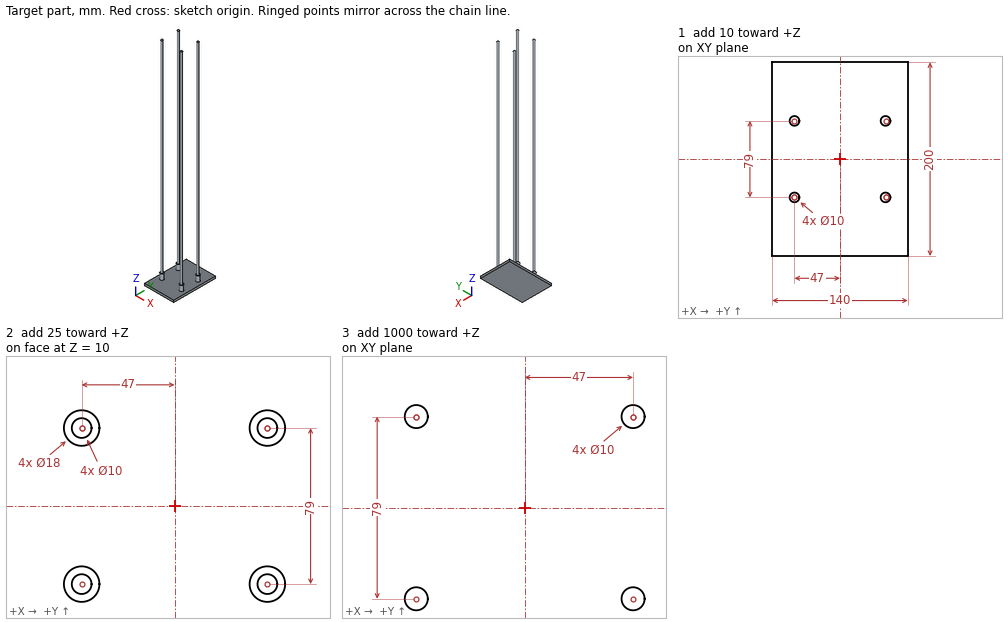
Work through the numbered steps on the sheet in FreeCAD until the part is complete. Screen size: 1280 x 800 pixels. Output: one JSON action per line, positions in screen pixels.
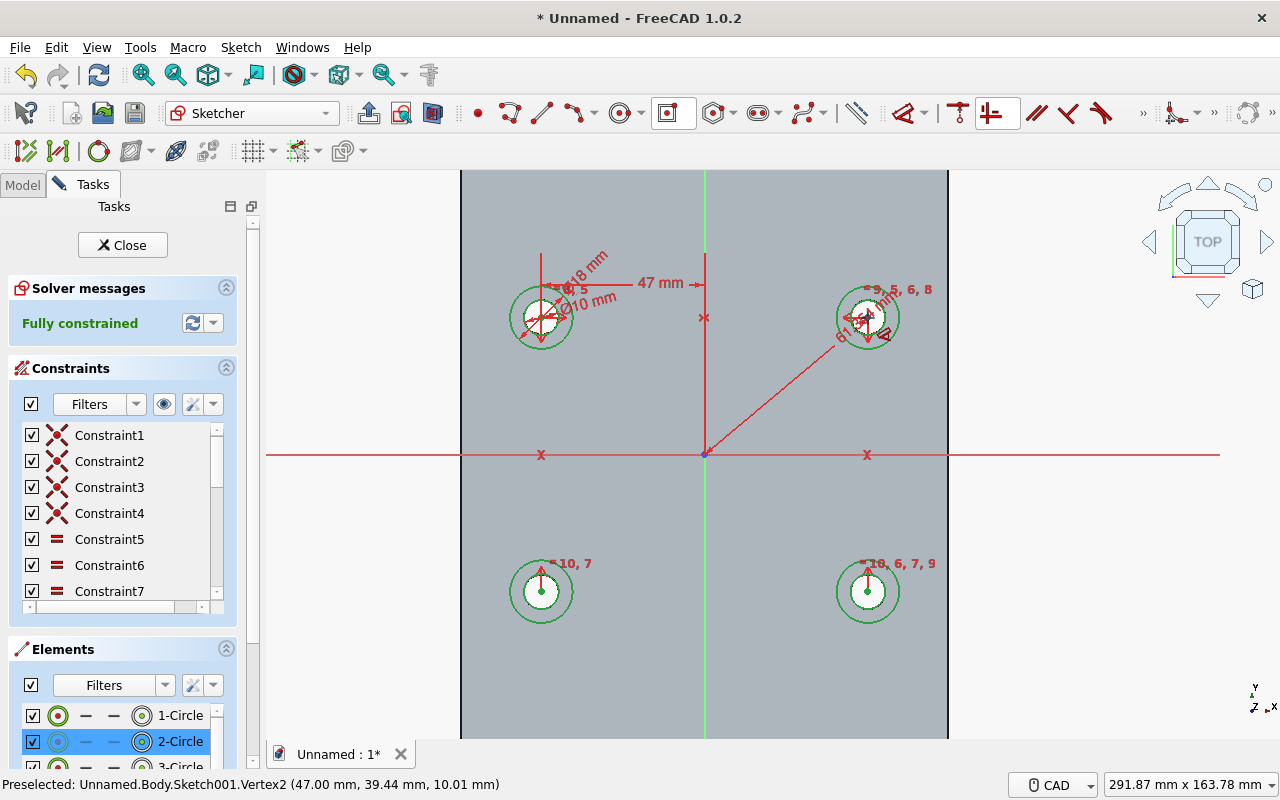
{"action": "left_click", "coordinate": [868, 592]}
{"action": "left_click", "coordinate": [902, 392]}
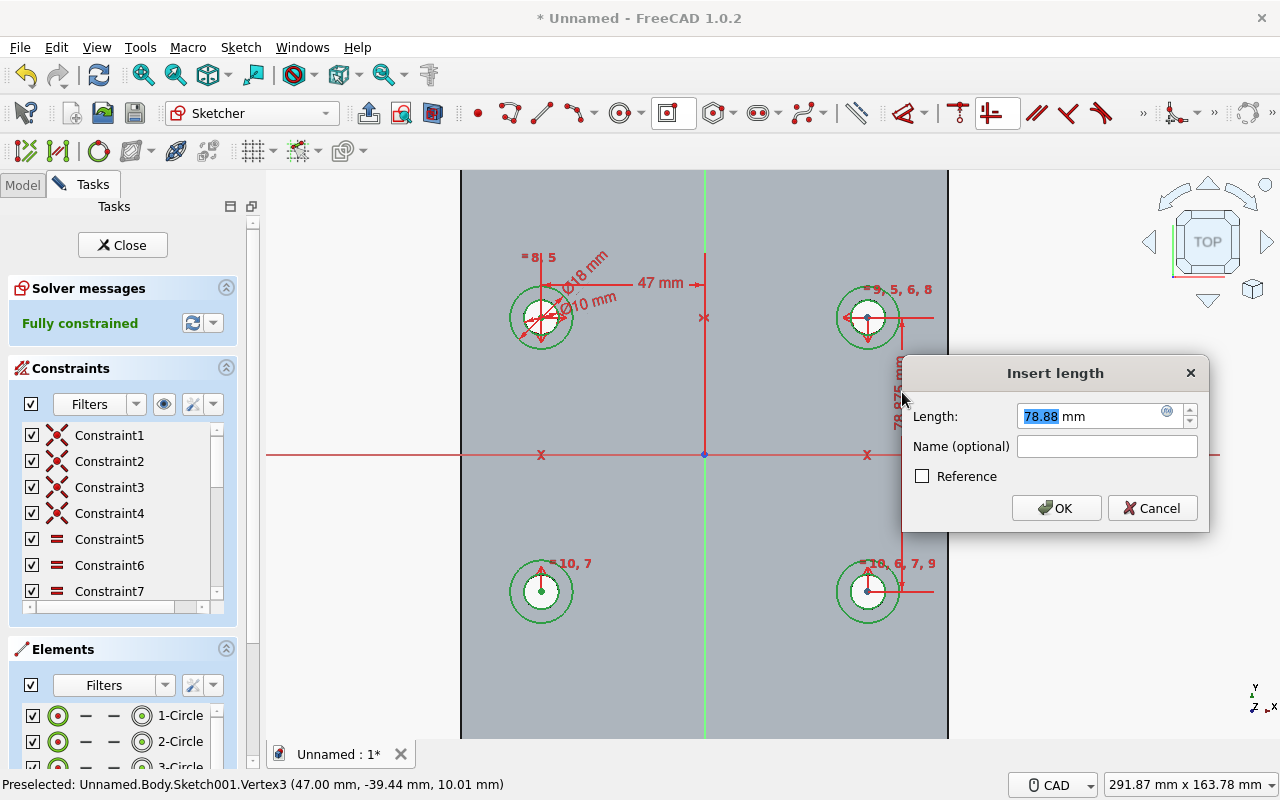
{"action": "type", "text": "79"}
{"action": "key", "text": "Return"}
{"action": "key", "text": "Escape"}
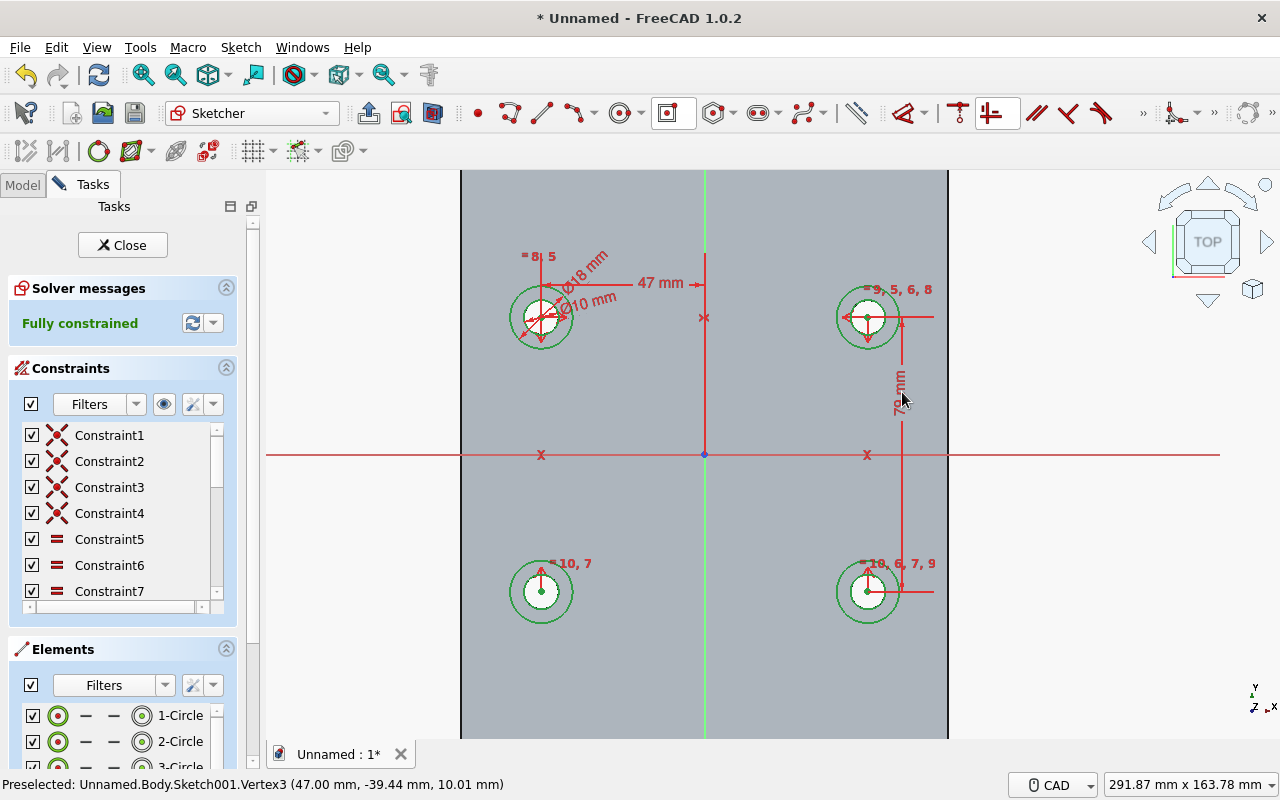
{"action": "left_click", "coordinate": [123, 245]}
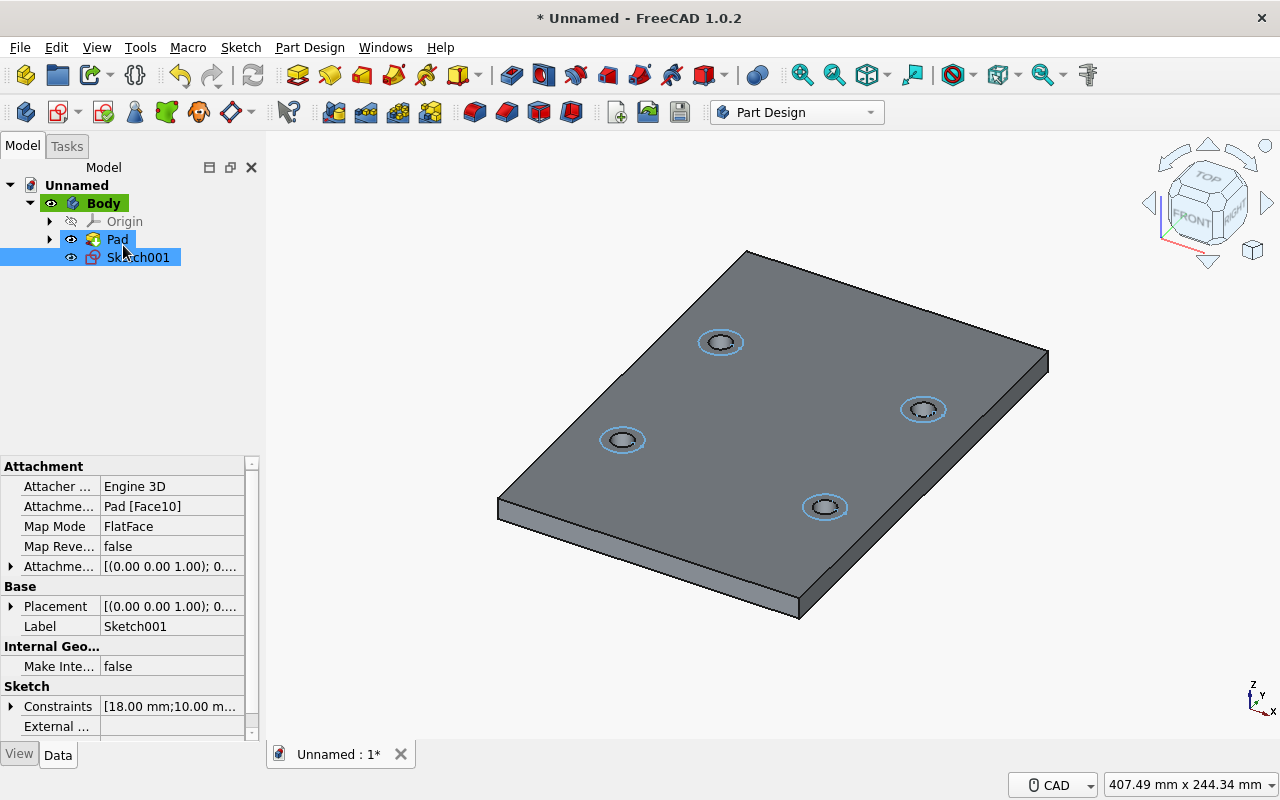
{"action": "left_click", "coordinate": [298, 76]}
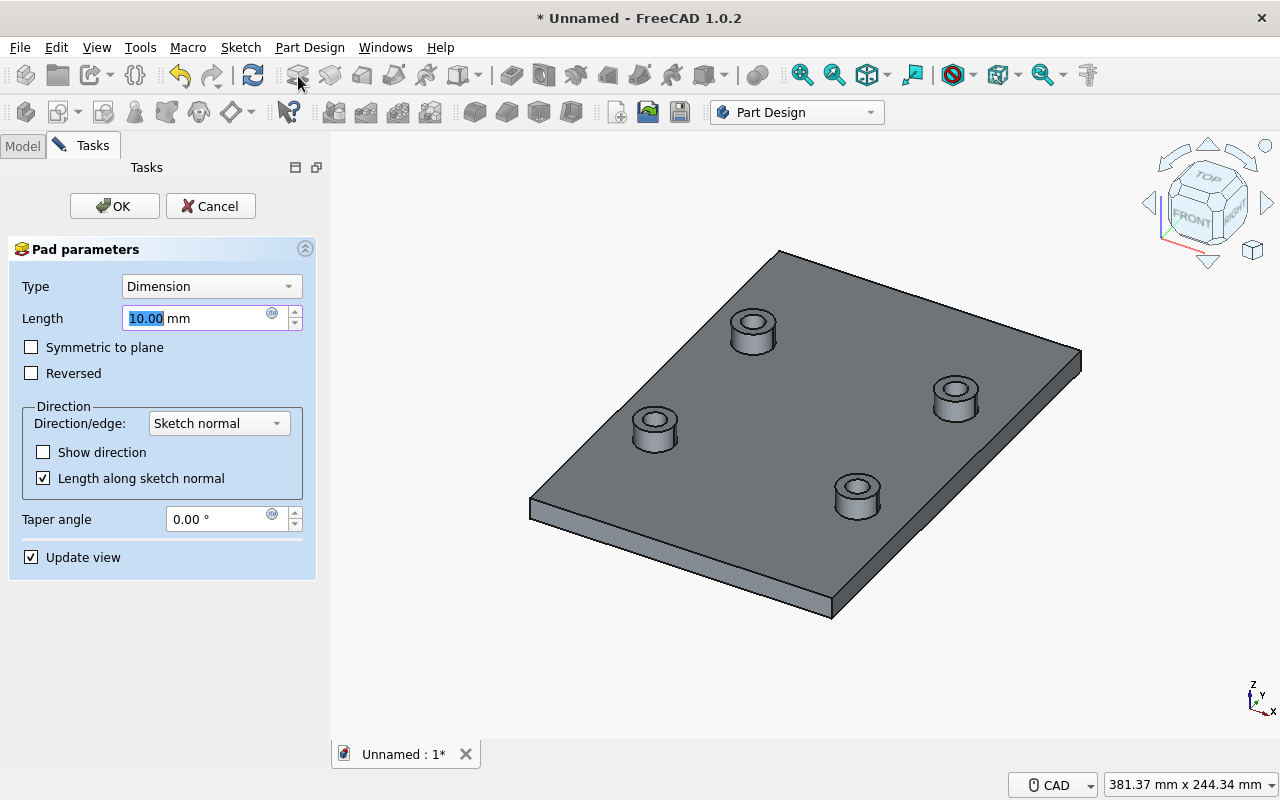
{"action": "type", "text": "25"}
{"action": "key", "text": "Tab"}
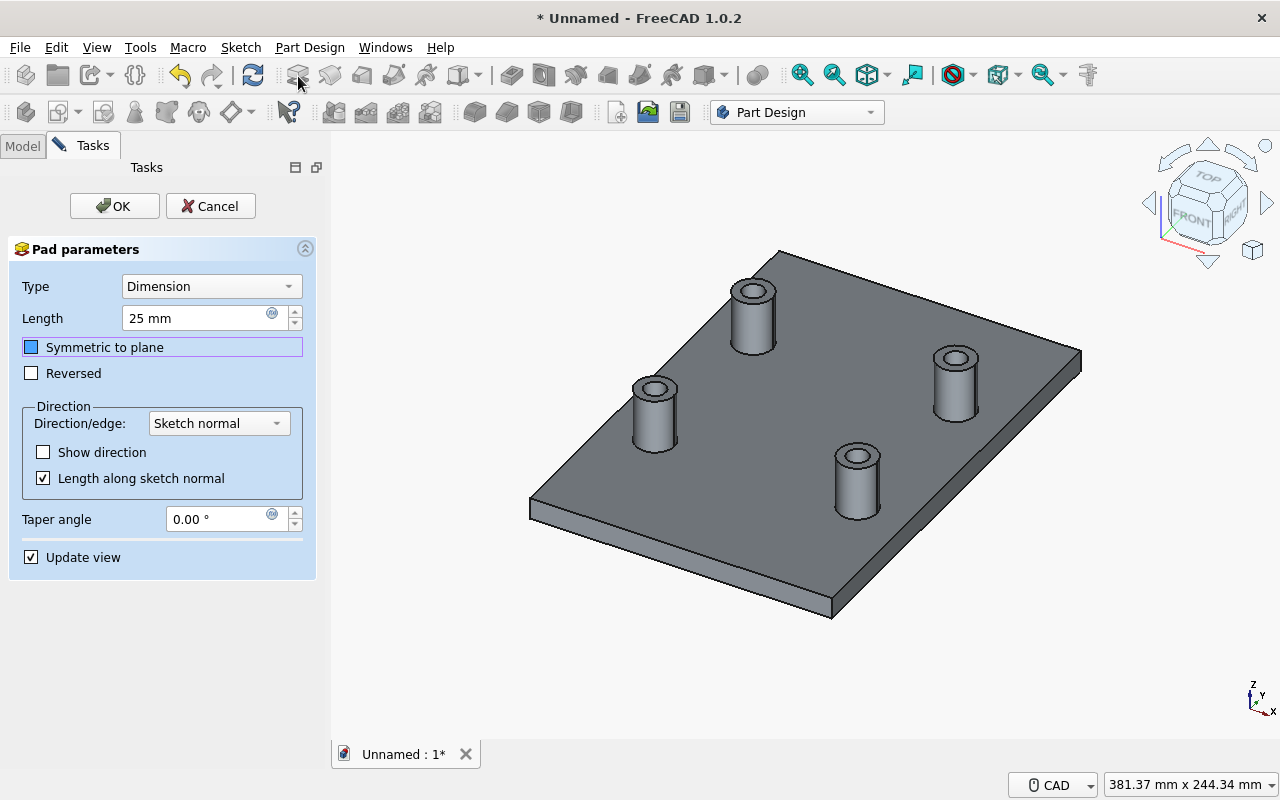
{"action": "left_click", "coordinate": [115, 206]}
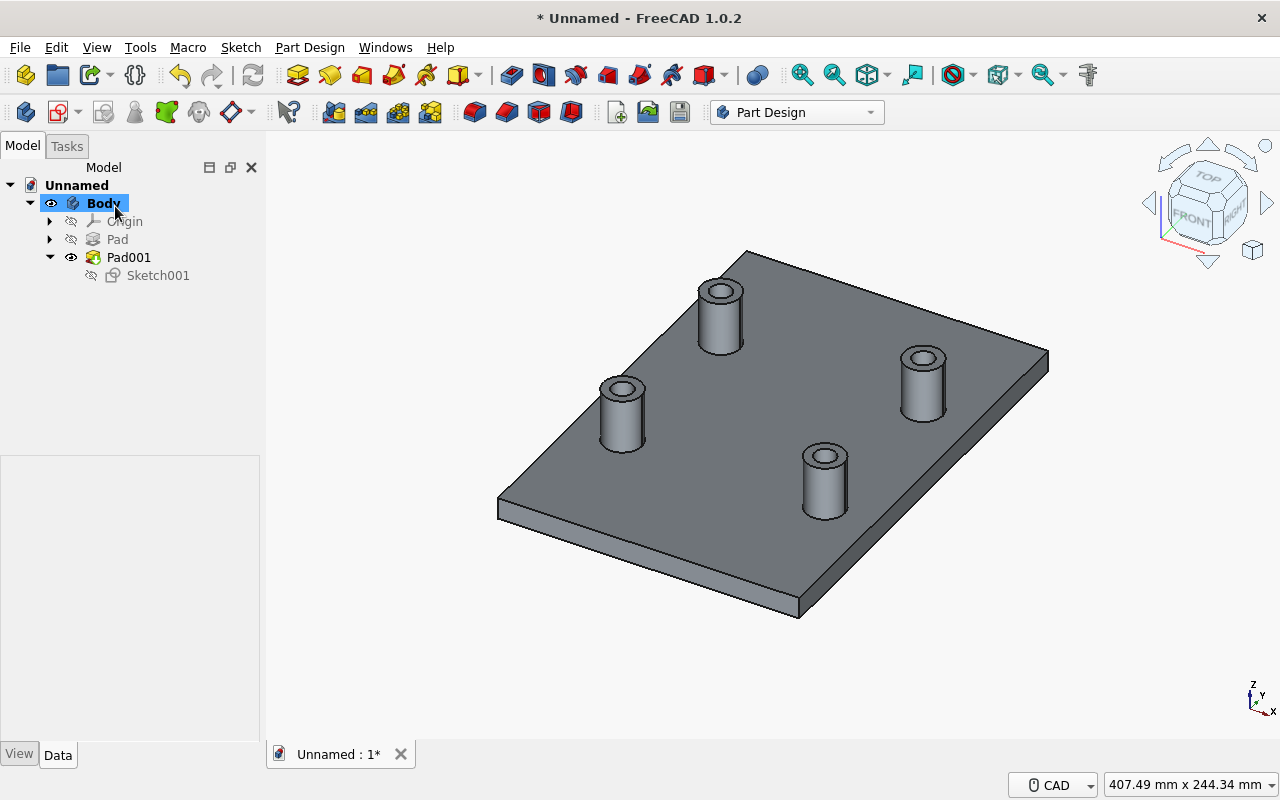
{"action": "left_click", "coordinate": [58, 112]}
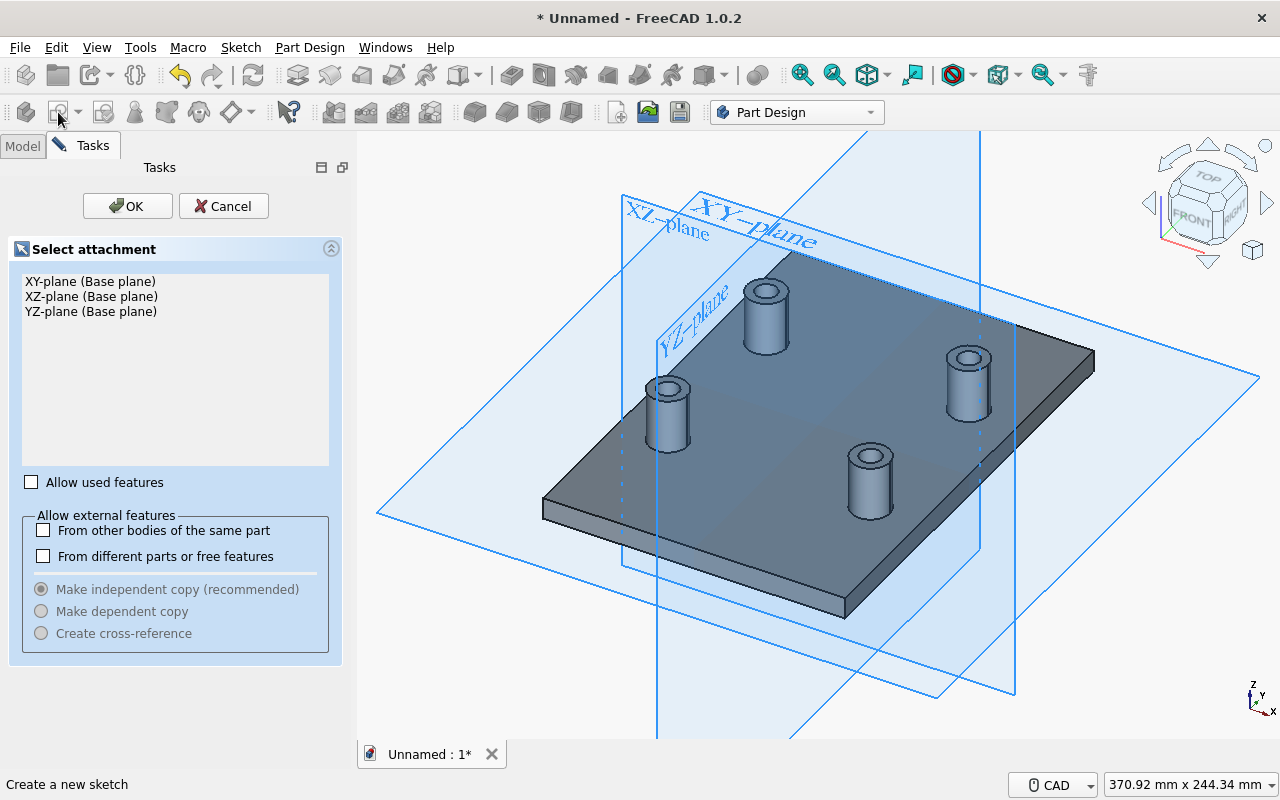
{"action": "left_click", "coordinate": [82, 282]}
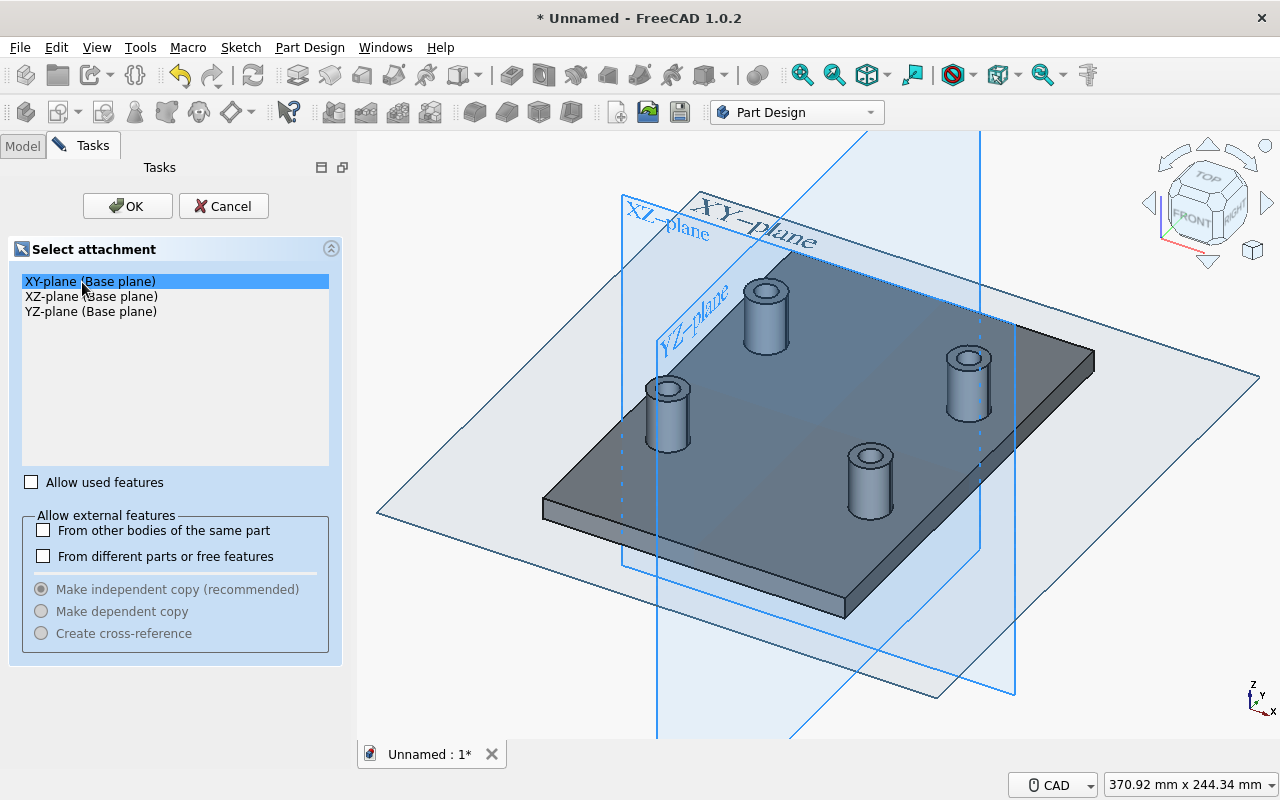
{"action": "left_click", "coordinate": [128, 206]}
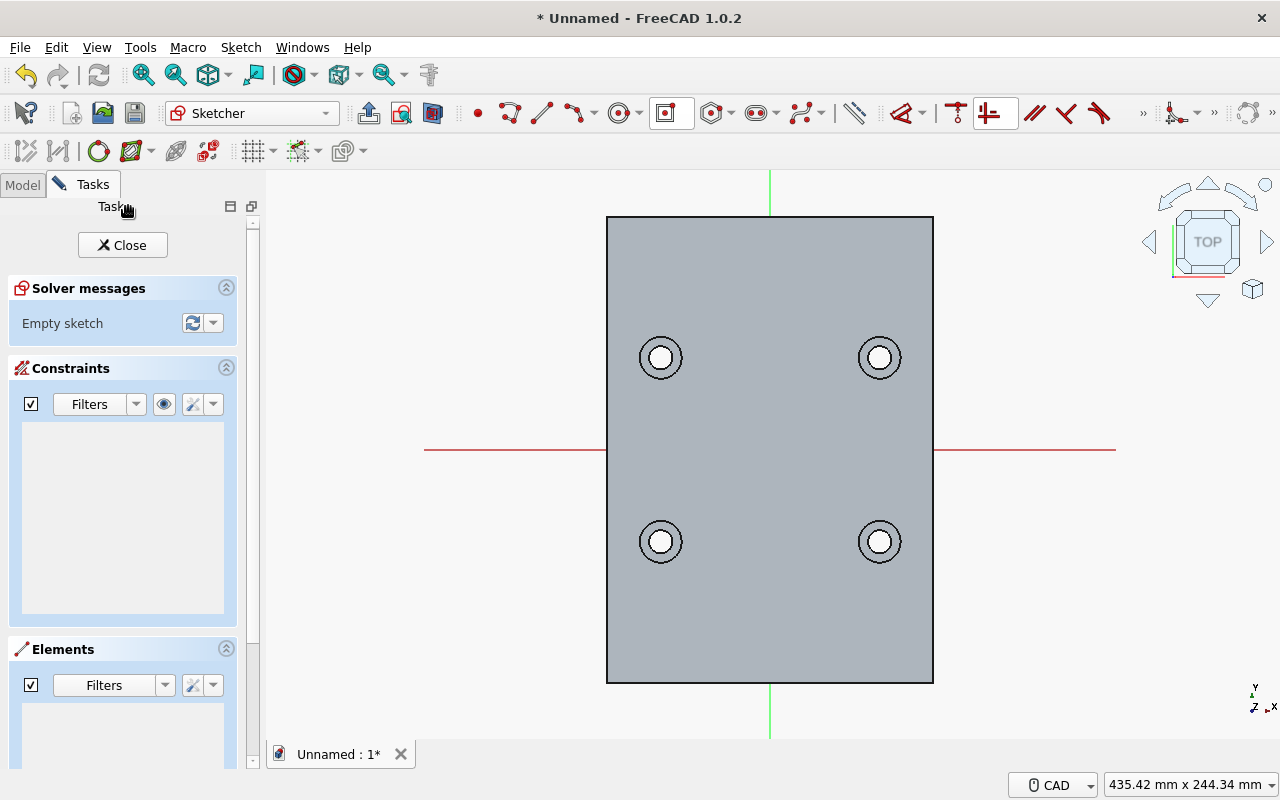
{"action": "left_click", "coordinate": [434, 114]}